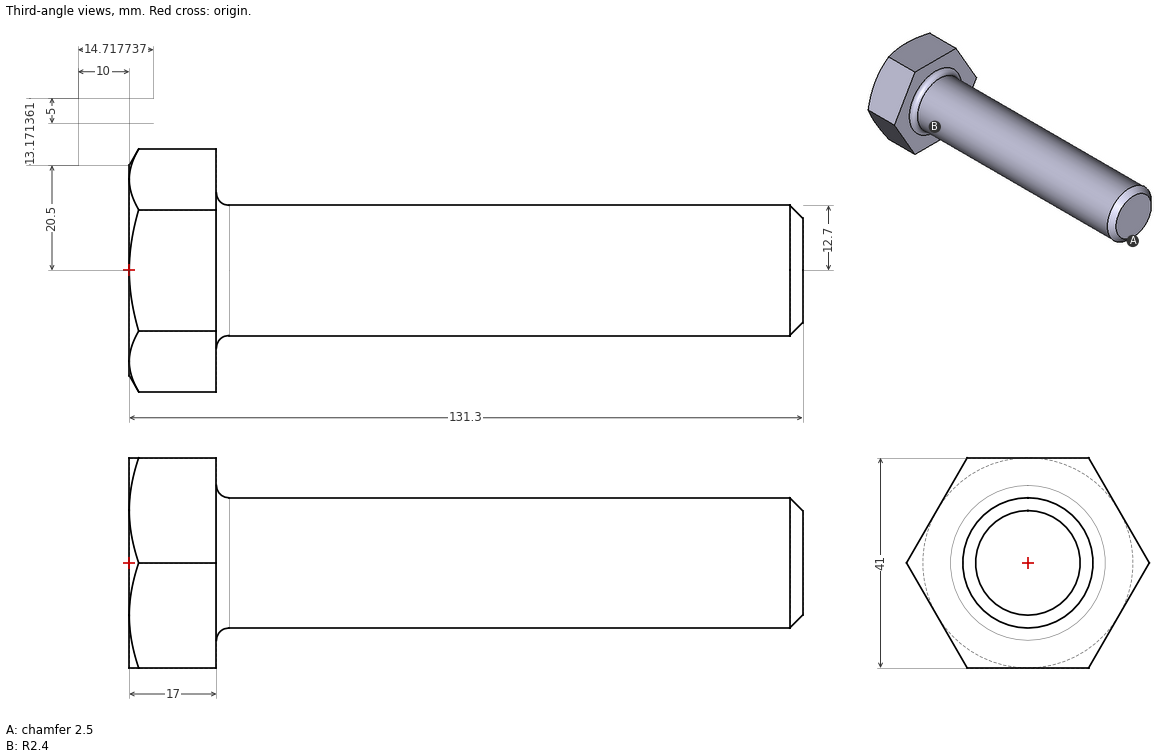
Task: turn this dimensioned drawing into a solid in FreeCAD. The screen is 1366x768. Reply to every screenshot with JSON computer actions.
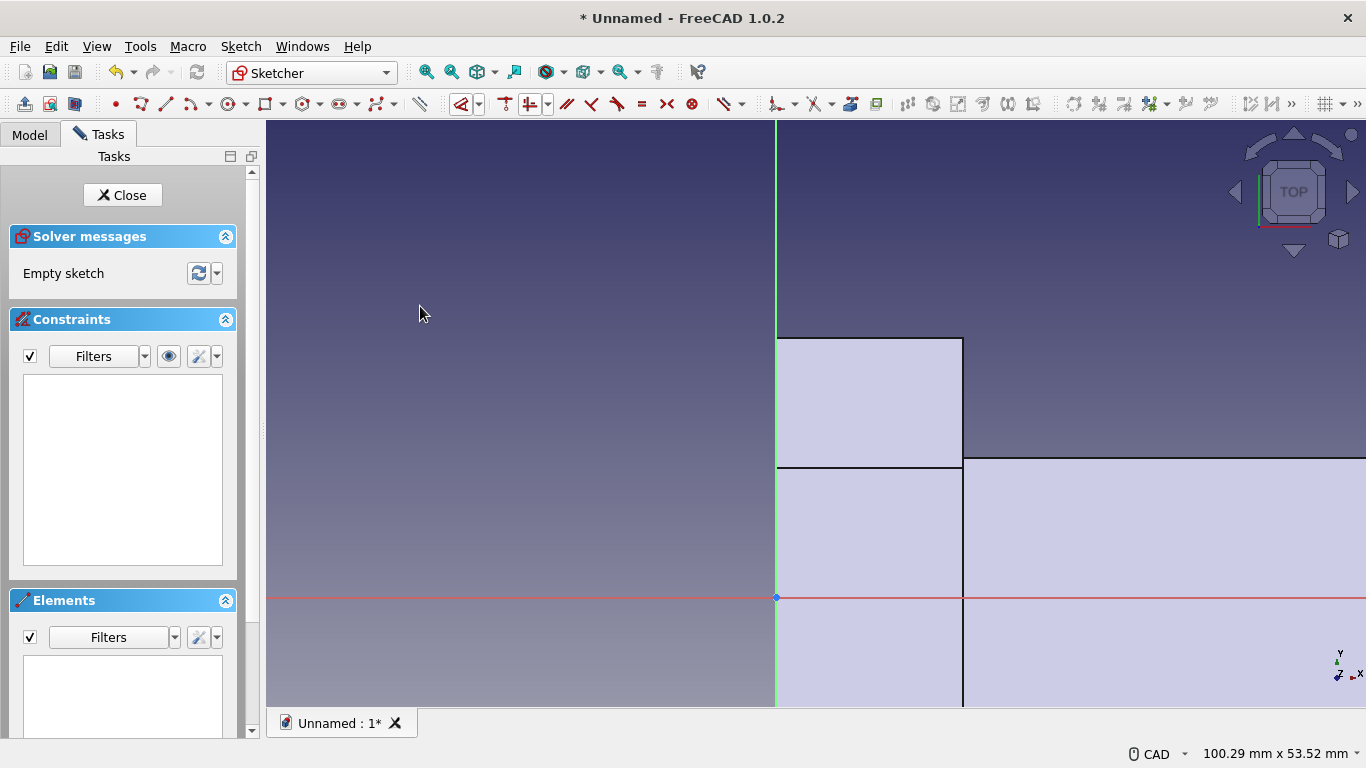
{"action": "left_click", "coordinate": [141, 104]}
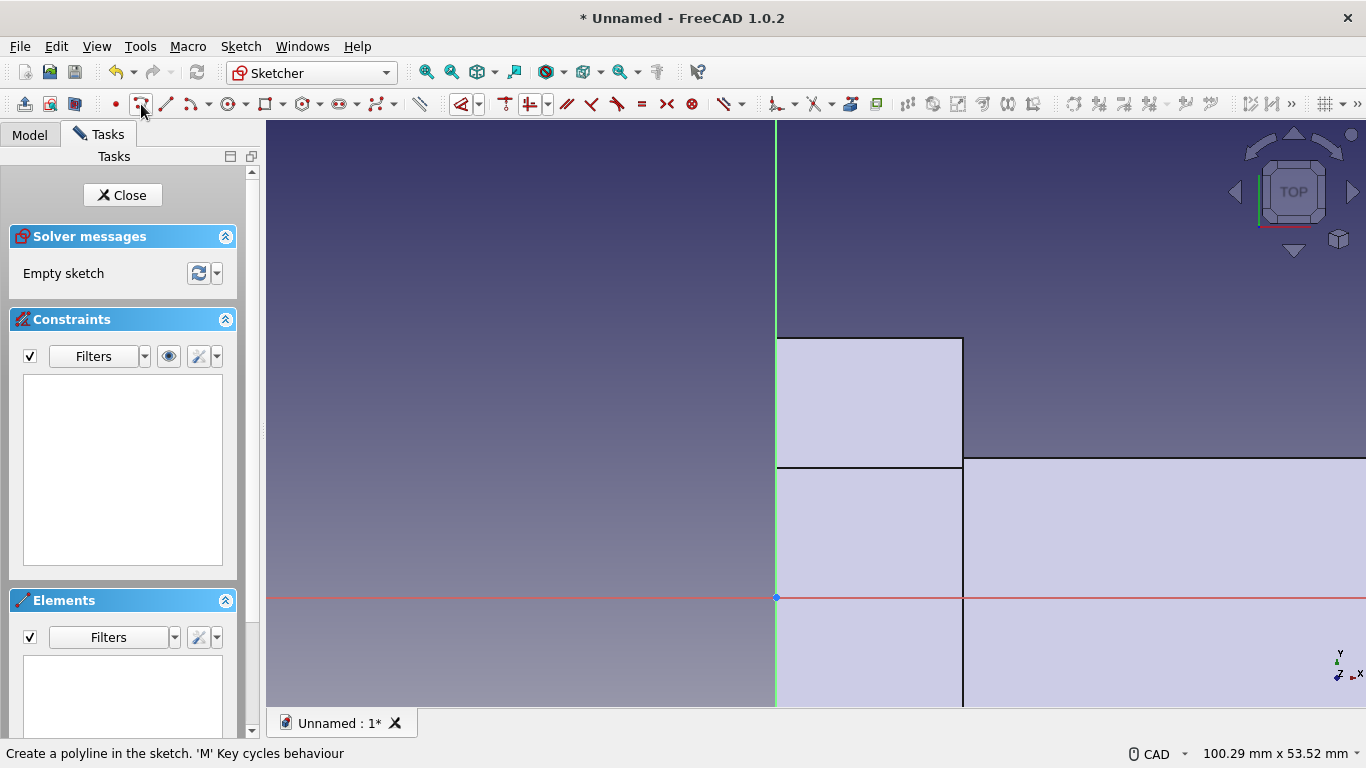
{"action": "left_click", "coordinate": [776, 373]}
{"action": "left_click", "coordinate": [828, 283]}
{"action": "left_click", "coordinate": [828, 228]}
{"action": "left_click", "coordinate": [666, 228]}
{"action": "left_click", "coordinate": [666, 373]}
{"action": "left_click", "coordinate": [776, 374]}
{"action": "key", "text": "Escape"}
{"action": "key", "text": "Escape"}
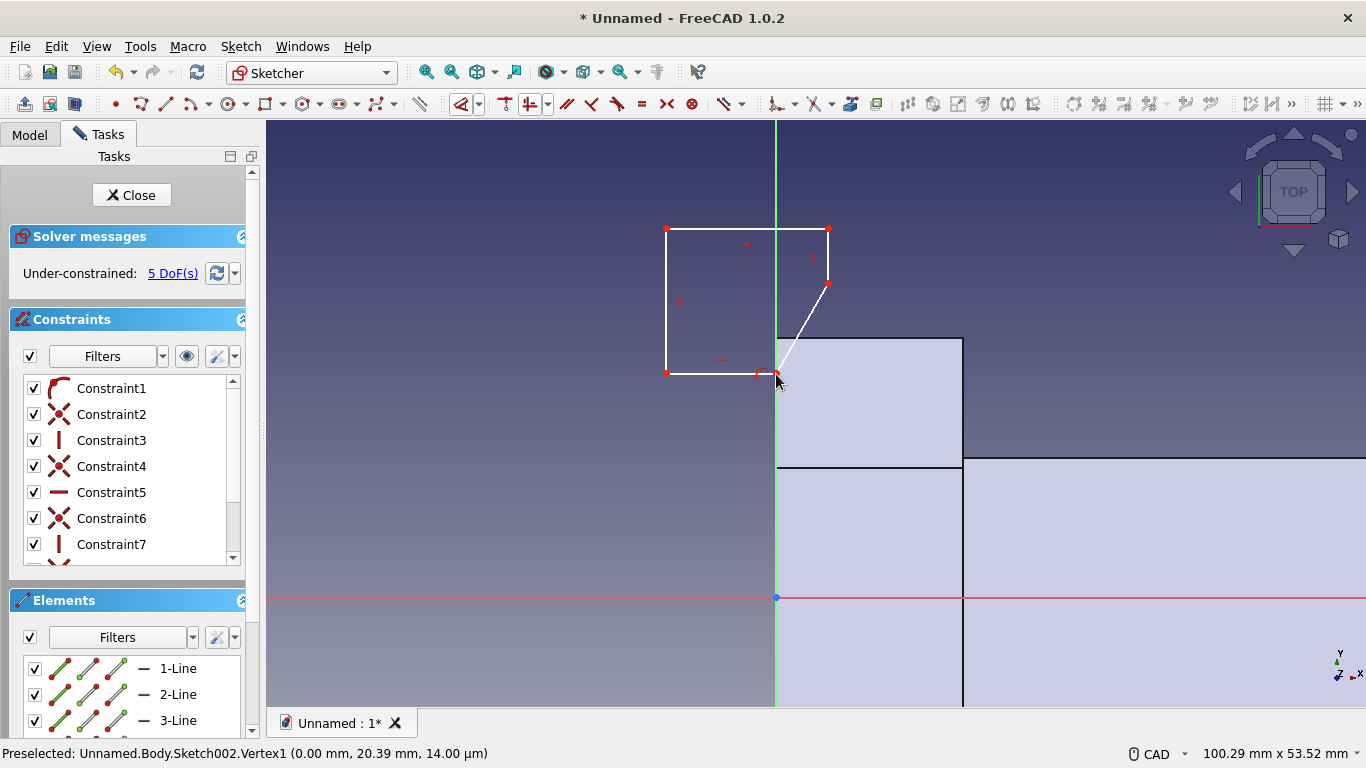
{"action": "key", "text": "d"}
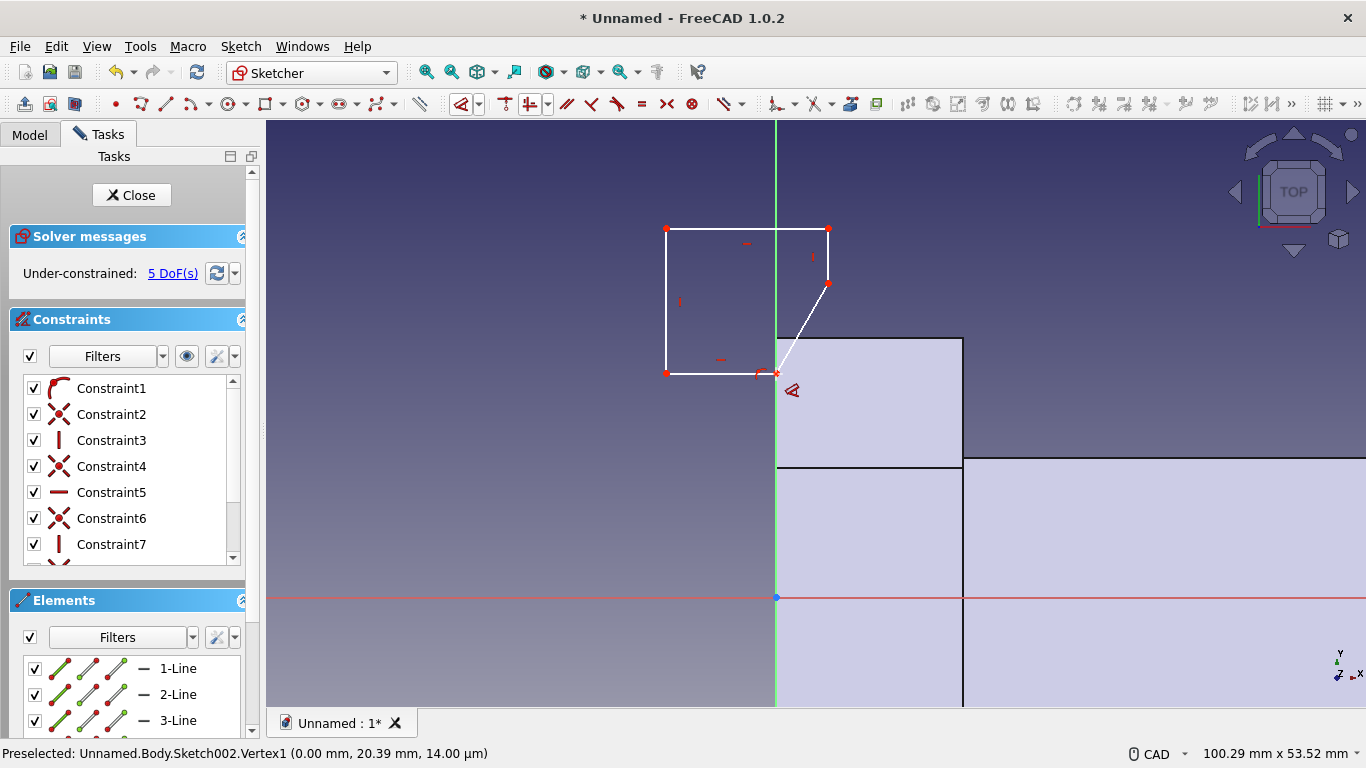
{"action": "left_click", "coordinate": [828, 267]}
{"action": "left_click", "coordinate": [862, 256]}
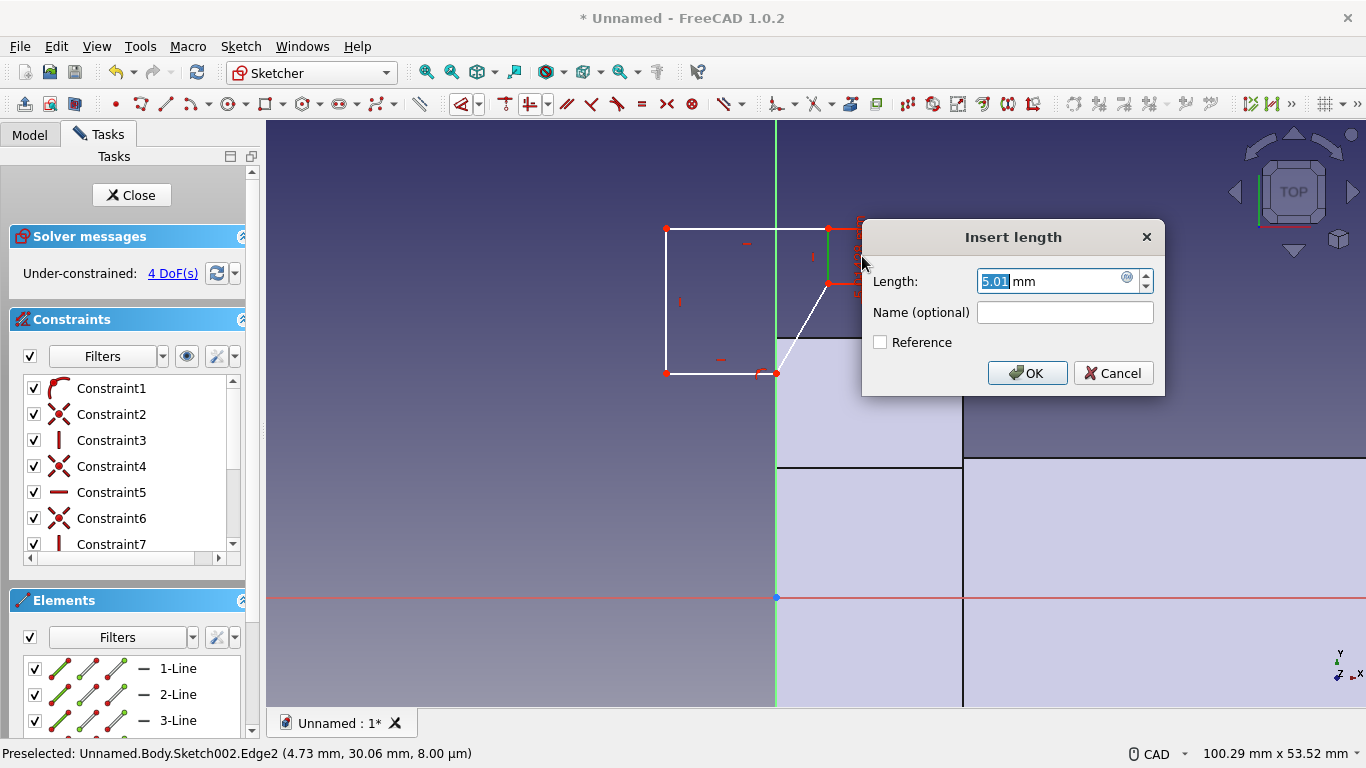
{"action": "type", "text": "5"}
{"action": "key", "text": "Return"}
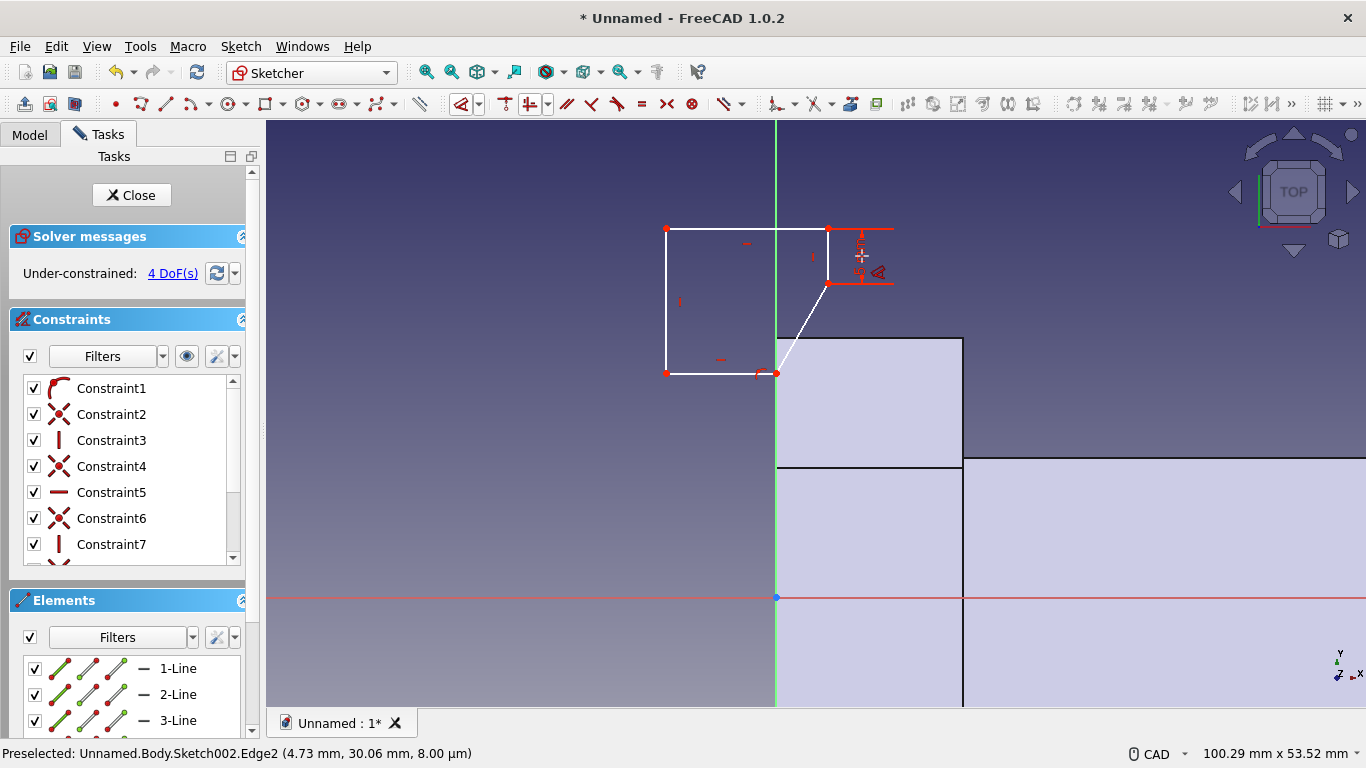
{"action": "left_click", "coordinate": [699, 374]}
{"action": "left_click", "coordinate": [721, 340]}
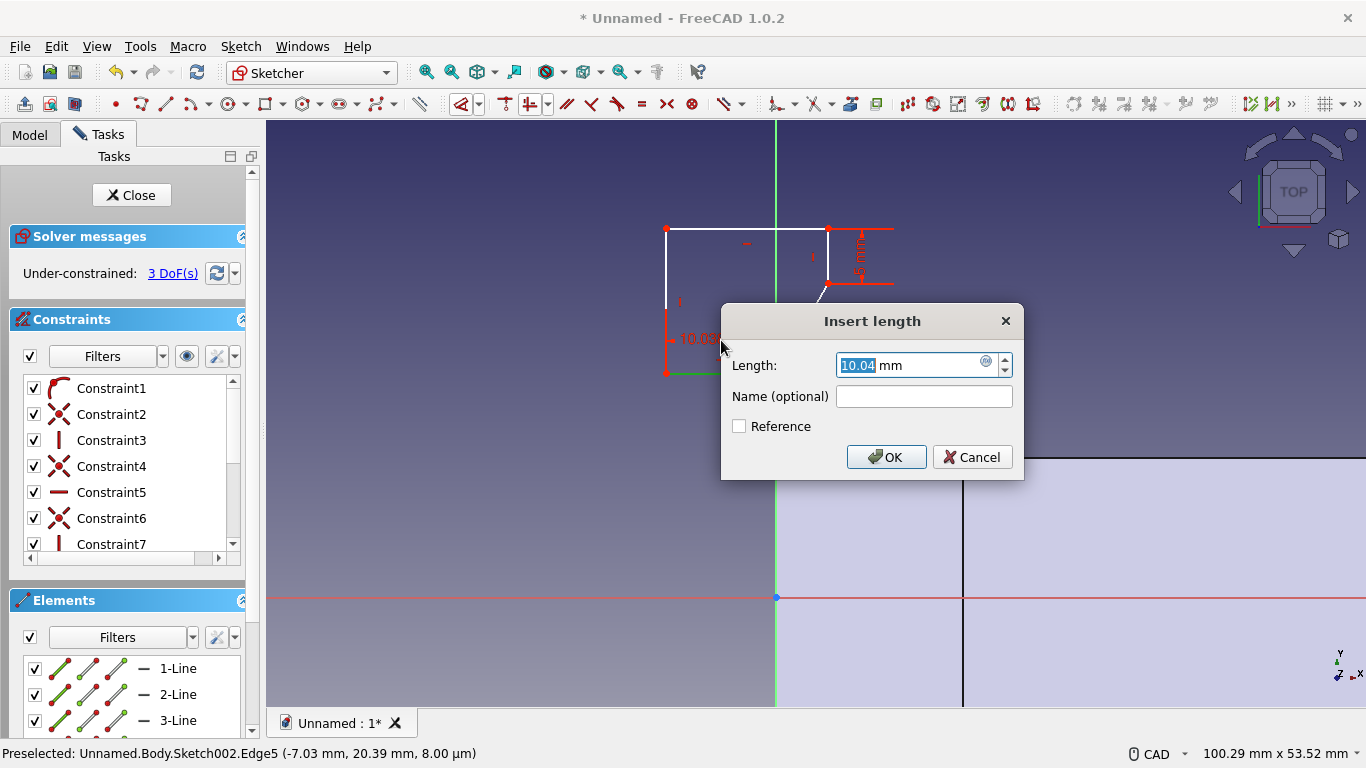
{"action": "type", "text": "10"}
{"action": "key", "text": "Return"}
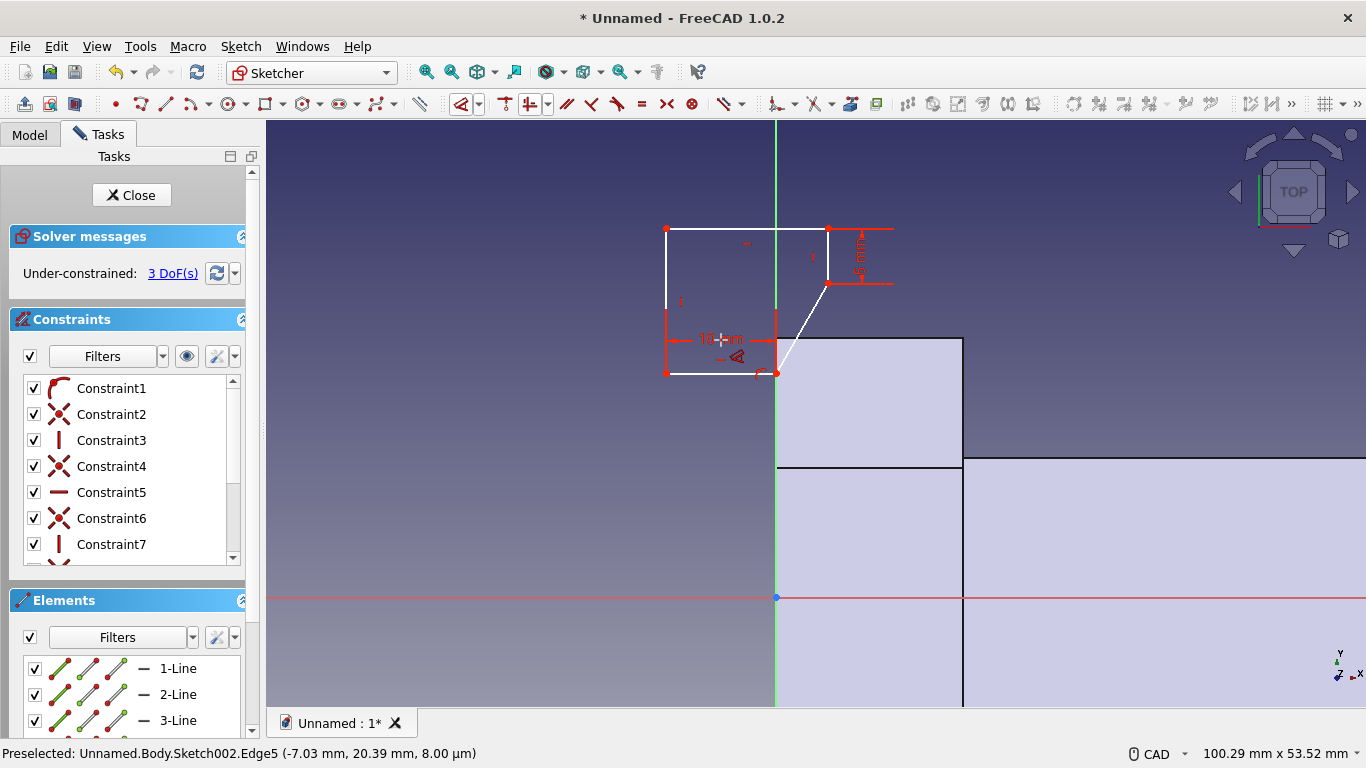
{"action": "left_click", "coordinate": [776, 374]}
{"action": "left_click", "coordinate": [810, 486]}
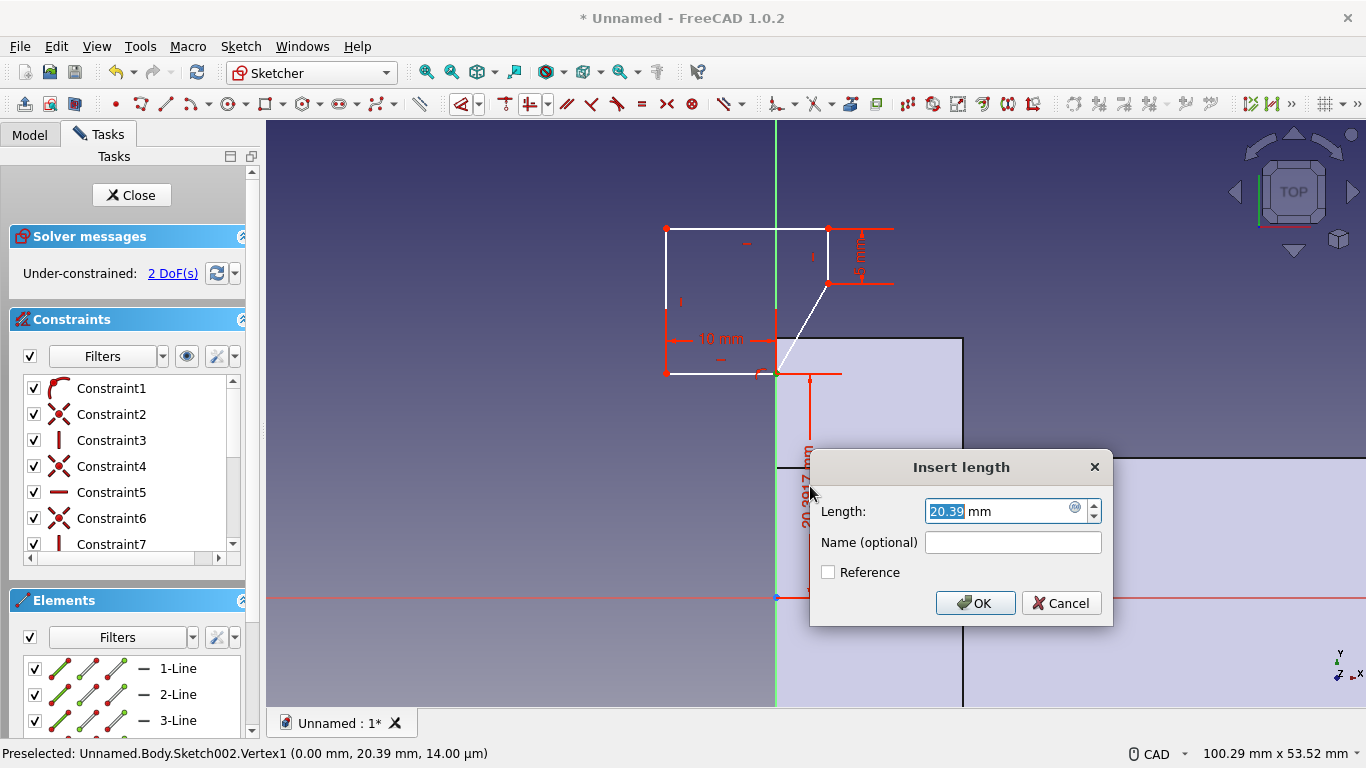
{"action": "type", "text": "20.5"}
{"action": "key", "text": "Return"}